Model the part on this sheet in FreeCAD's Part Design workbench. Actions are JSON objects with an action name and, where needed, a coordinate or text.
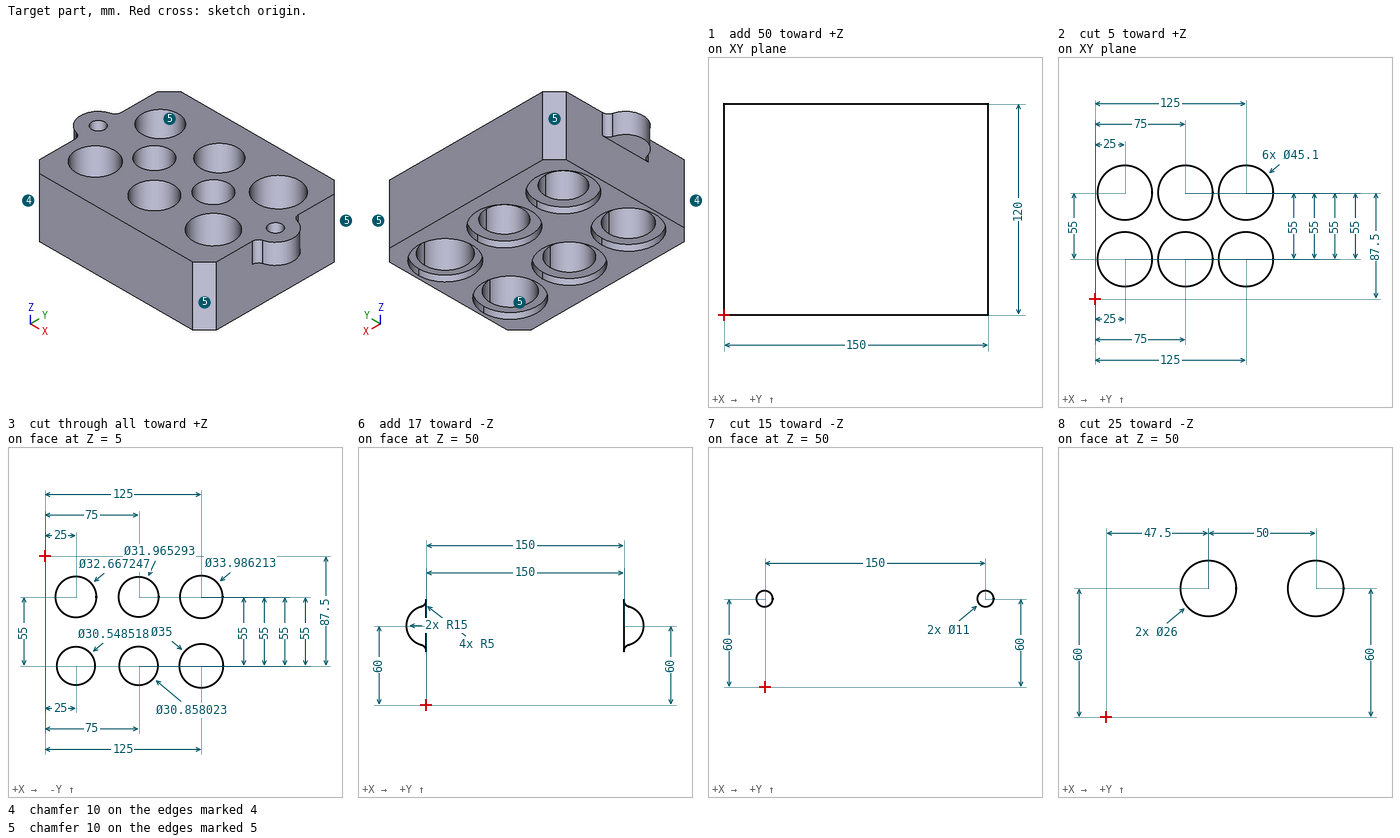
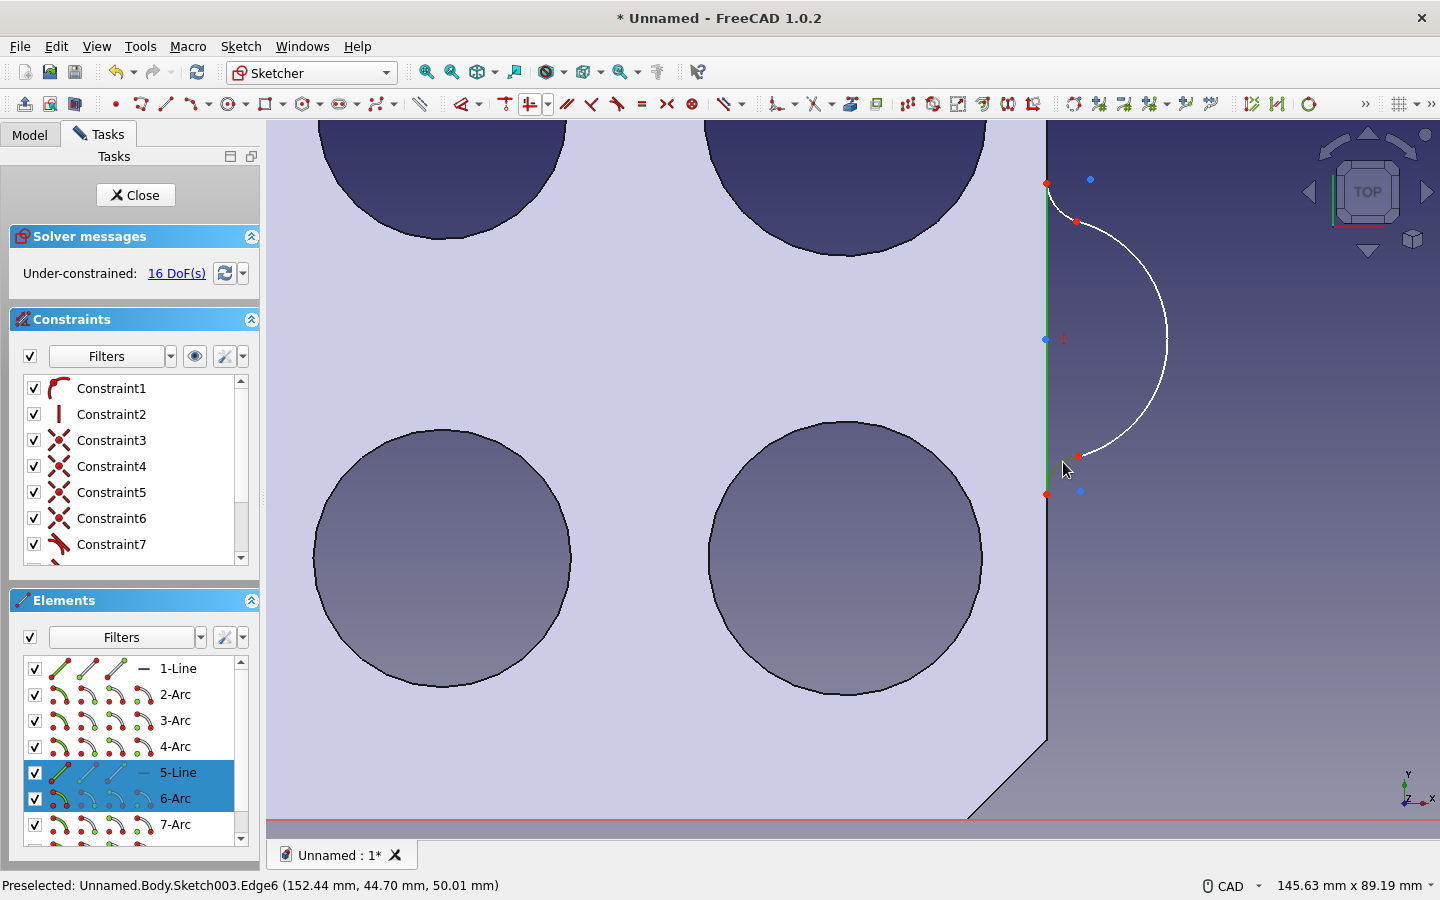
{"action": "key", "text": "t"}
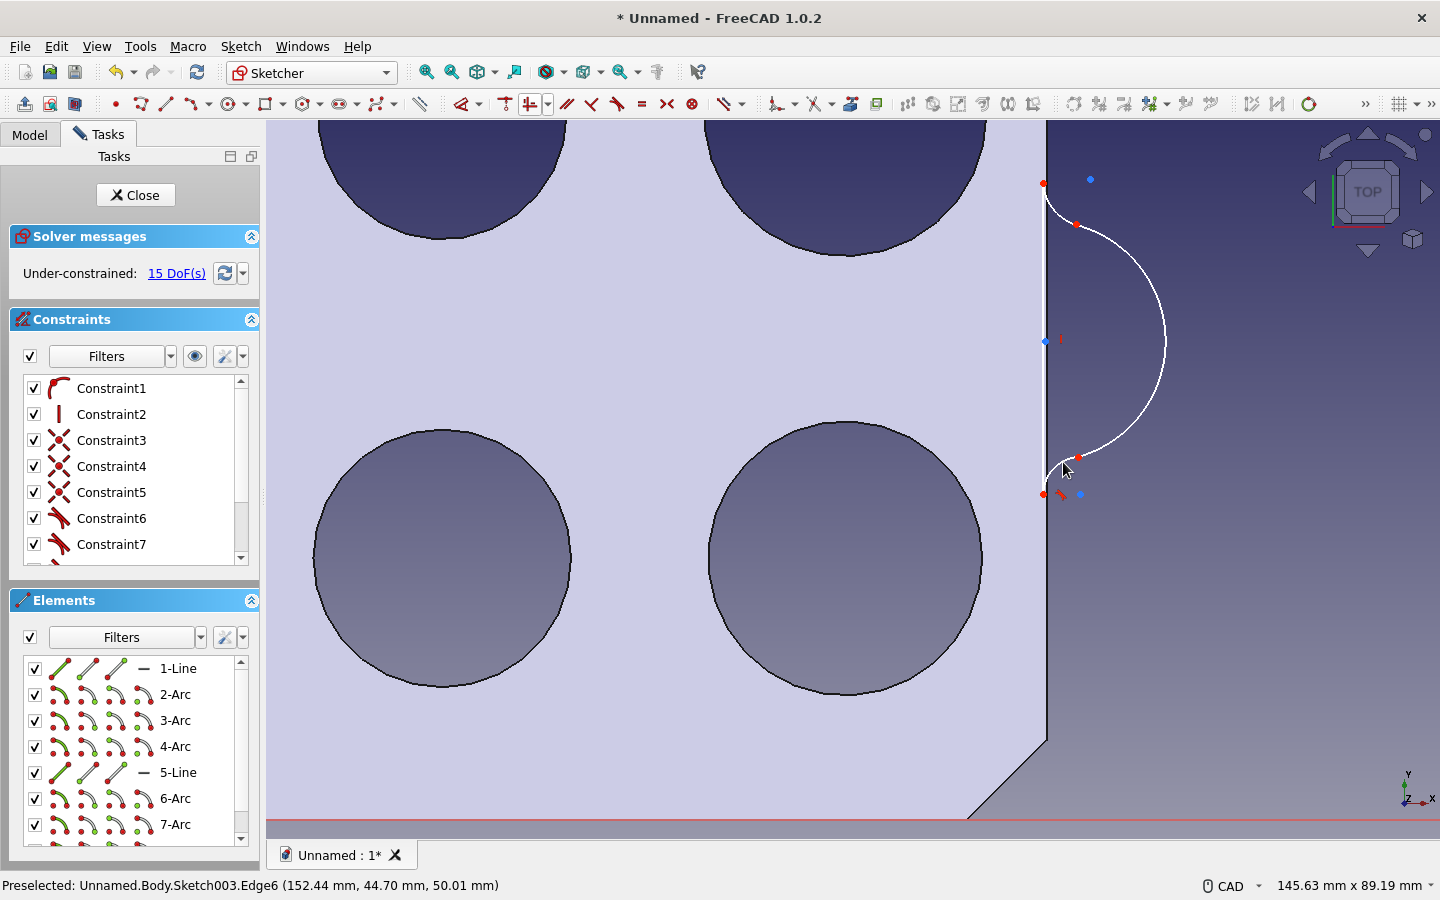
{"action": "left_click", "coordinate": [1043, 277]}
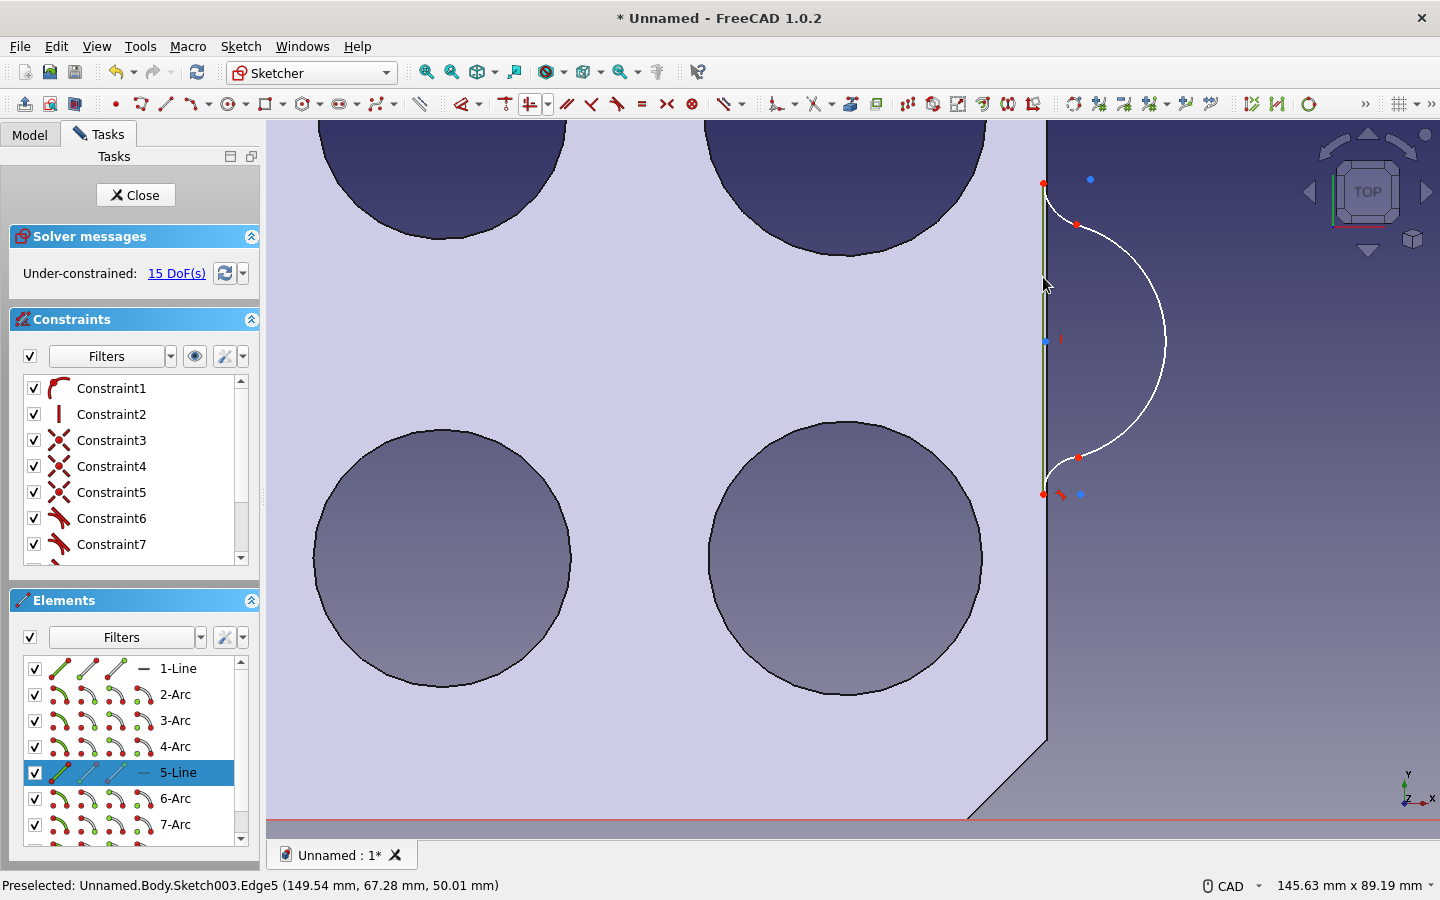
{"action": "left_click", "coordinate": [1061, 217]}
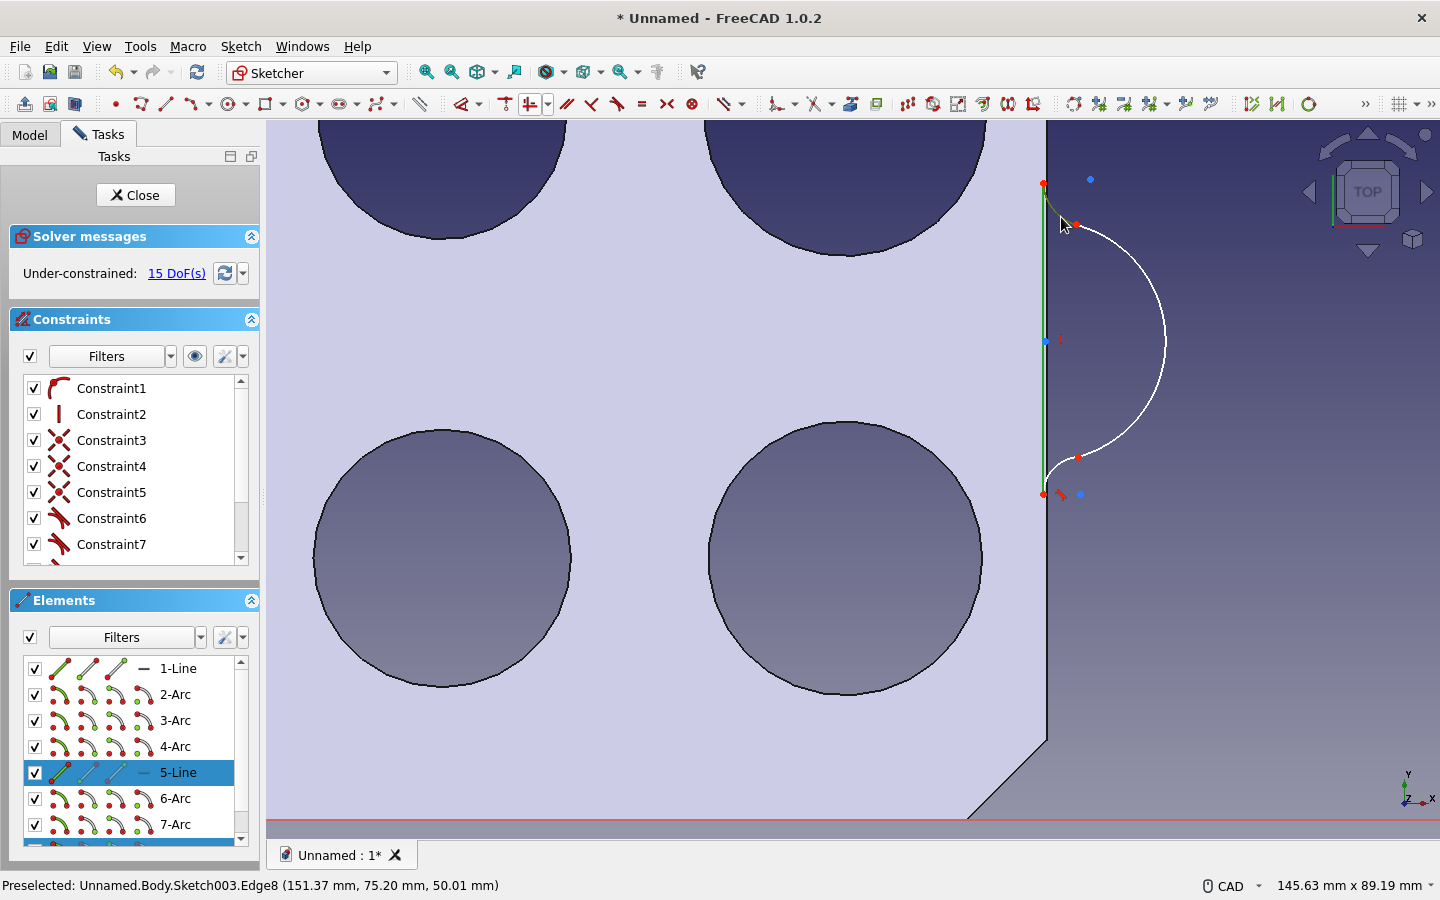
{"action": "left_click", "coordinate": [617, 104]}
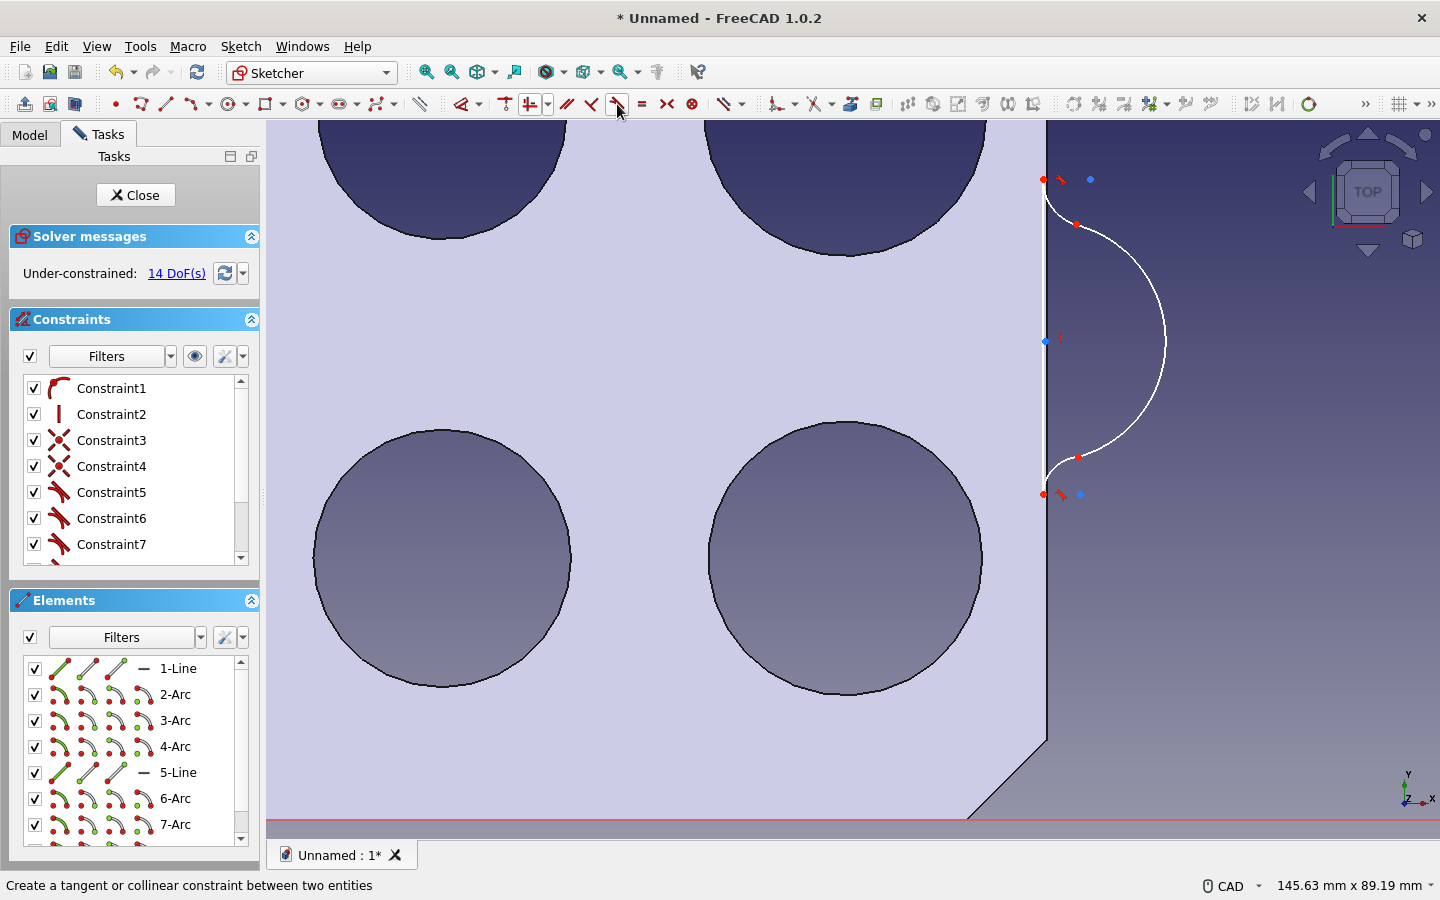
{"action": "left_click", "coordinate": [1062, 462]}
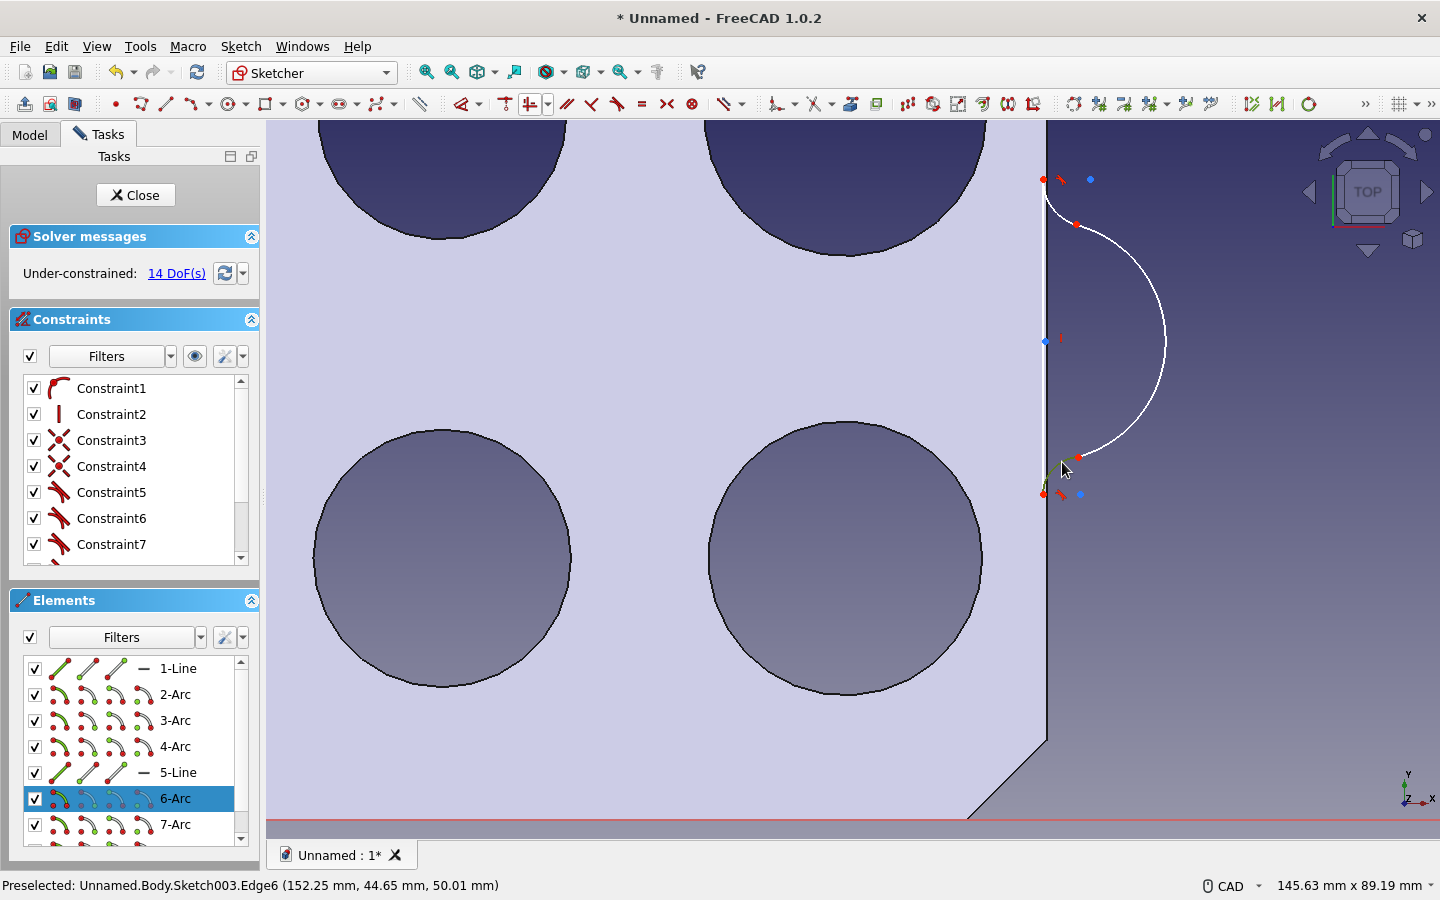
{"action": "left_click", "coordinate": [1150, 400]}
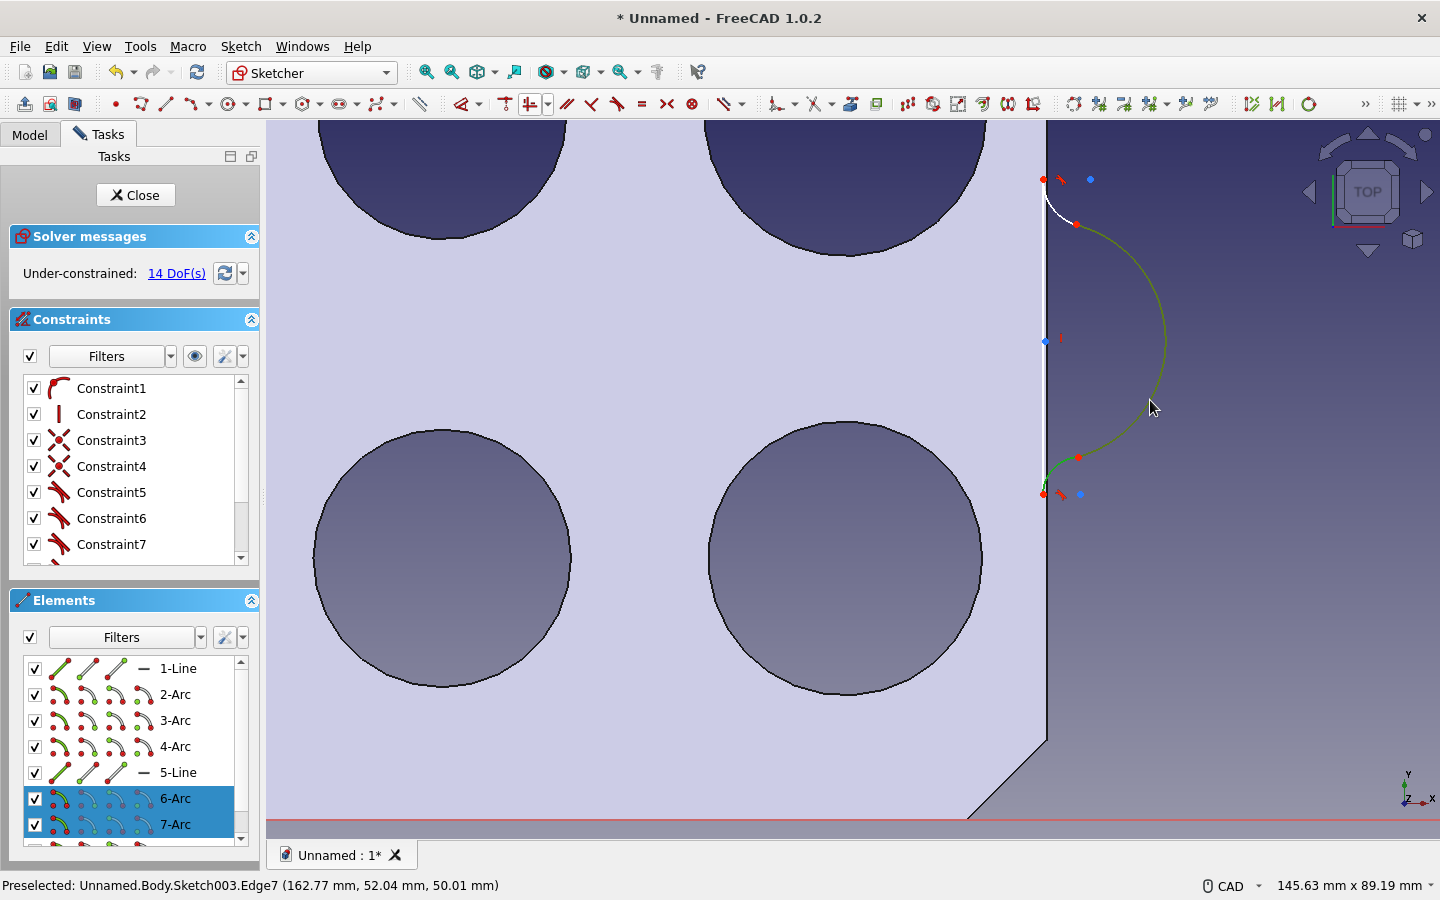
{"action": "left_click", "coordinate": [617, 104]}